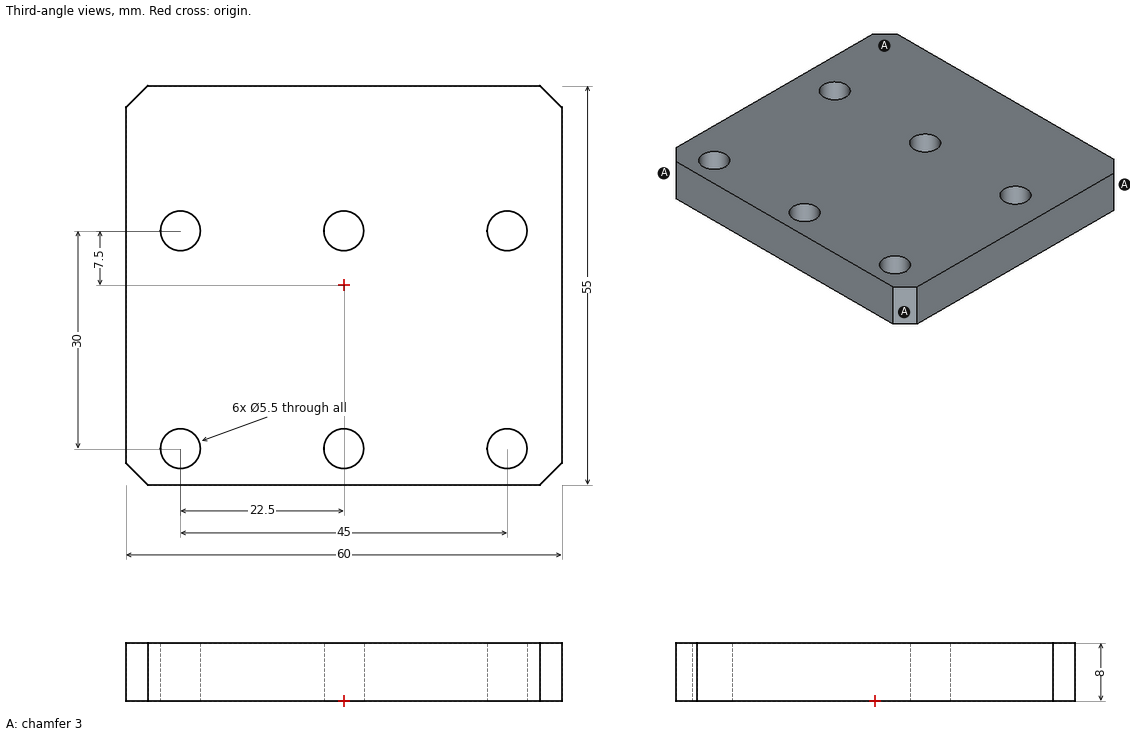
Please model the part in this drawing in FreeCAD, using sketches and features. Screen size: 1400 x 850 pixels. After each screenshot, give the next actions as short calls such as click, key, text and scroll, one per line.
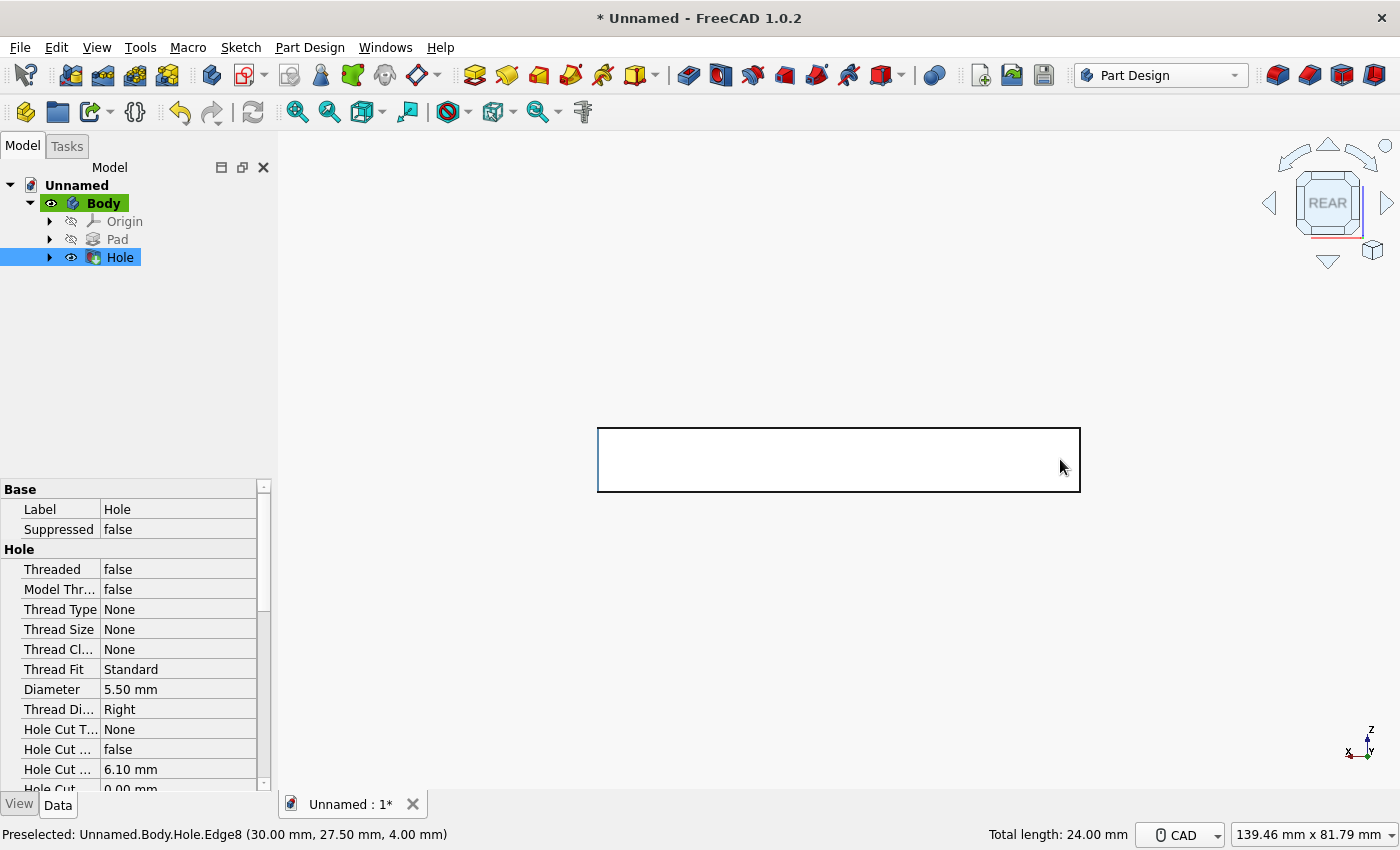
click(298, 112)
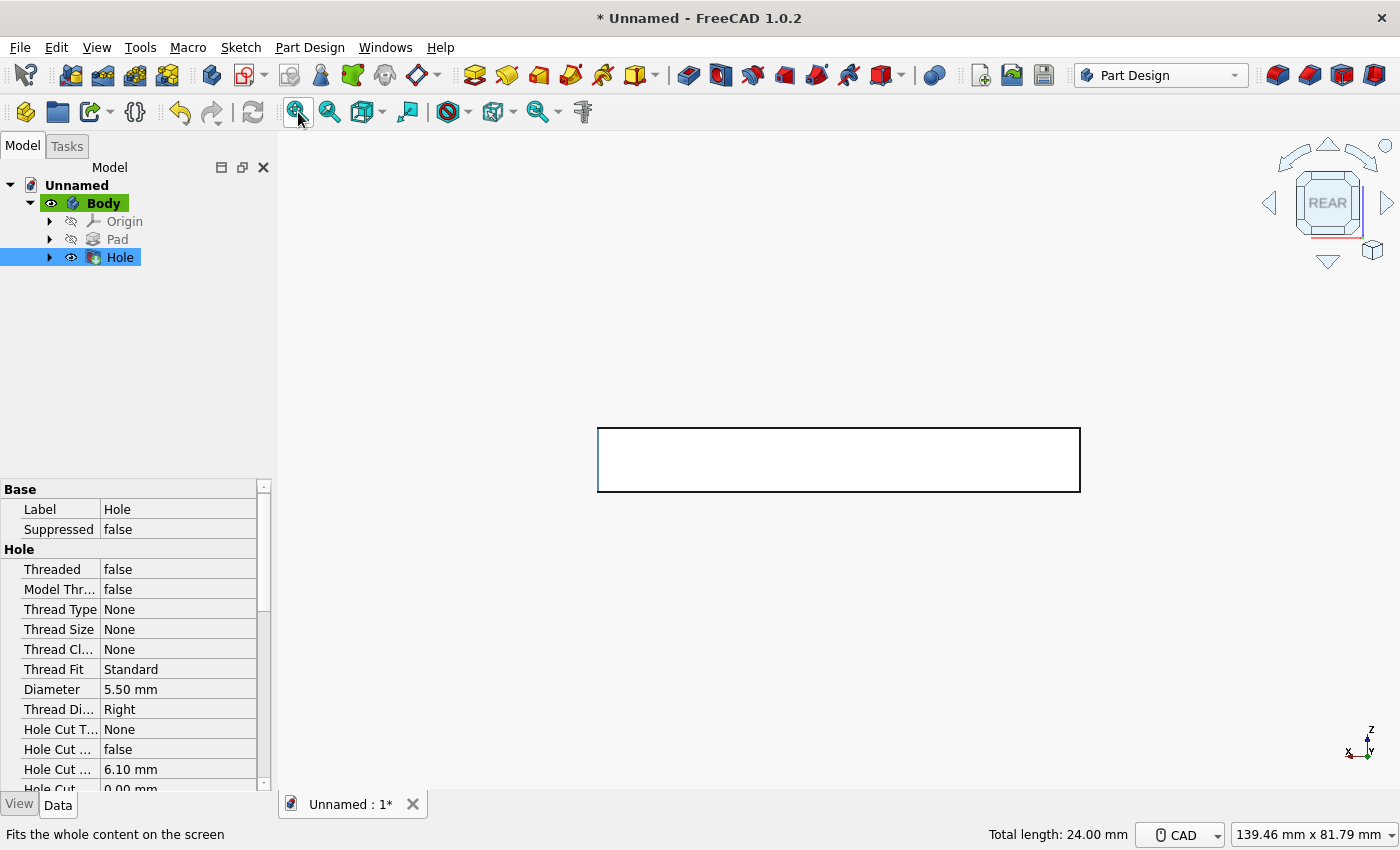
click(1080, 459, ctrl)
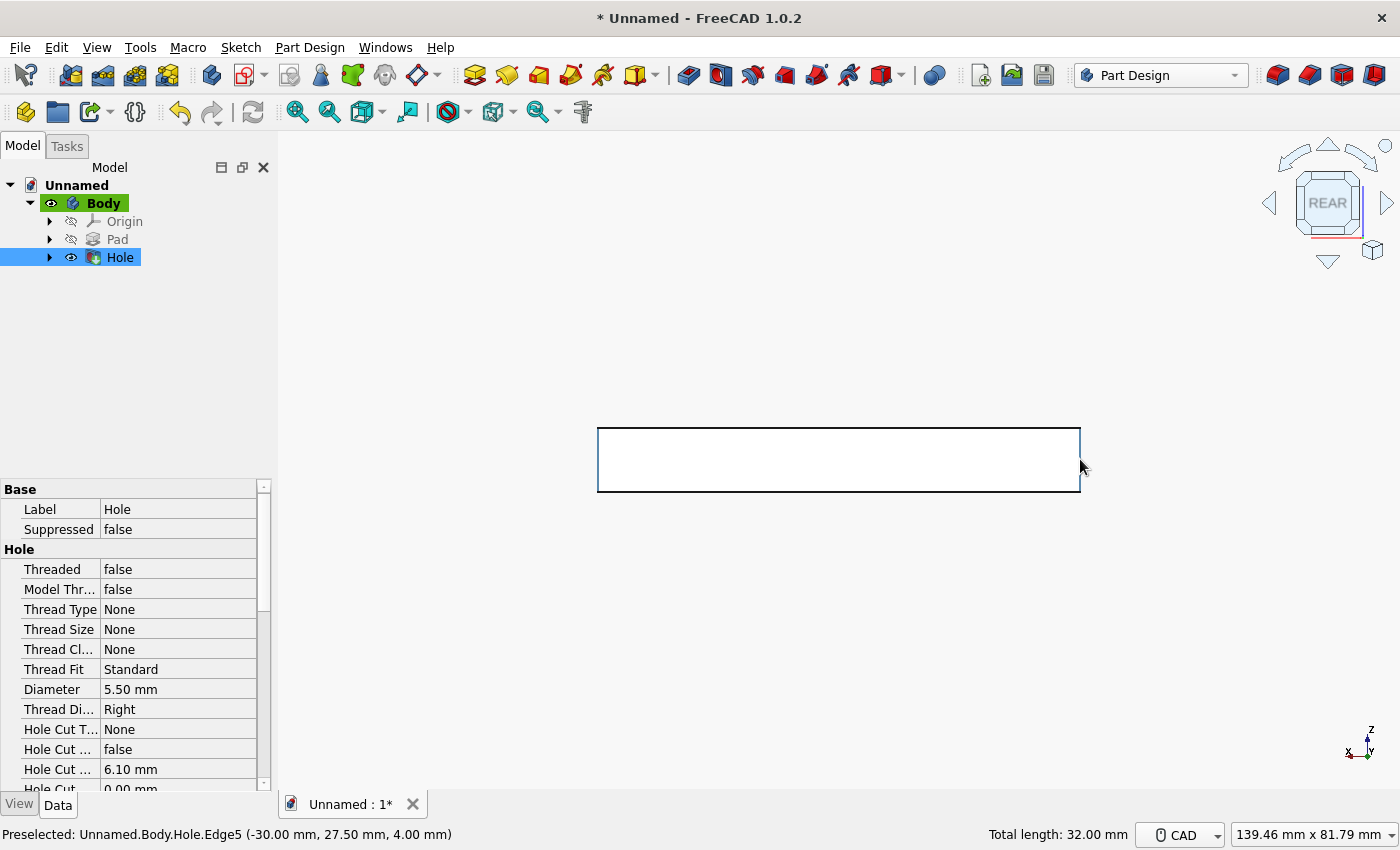
click(1310, 76)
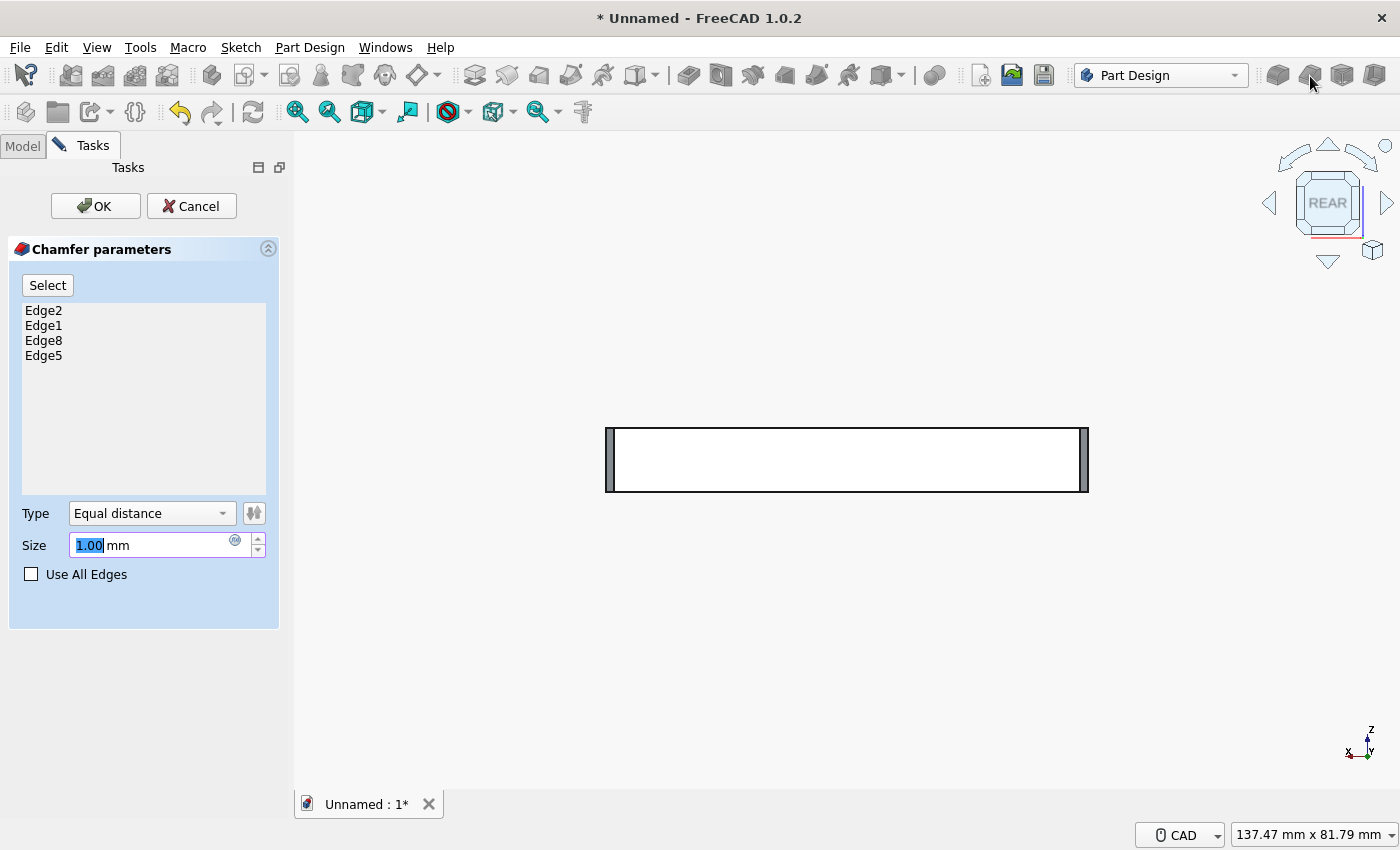
text(3)
key(Tab)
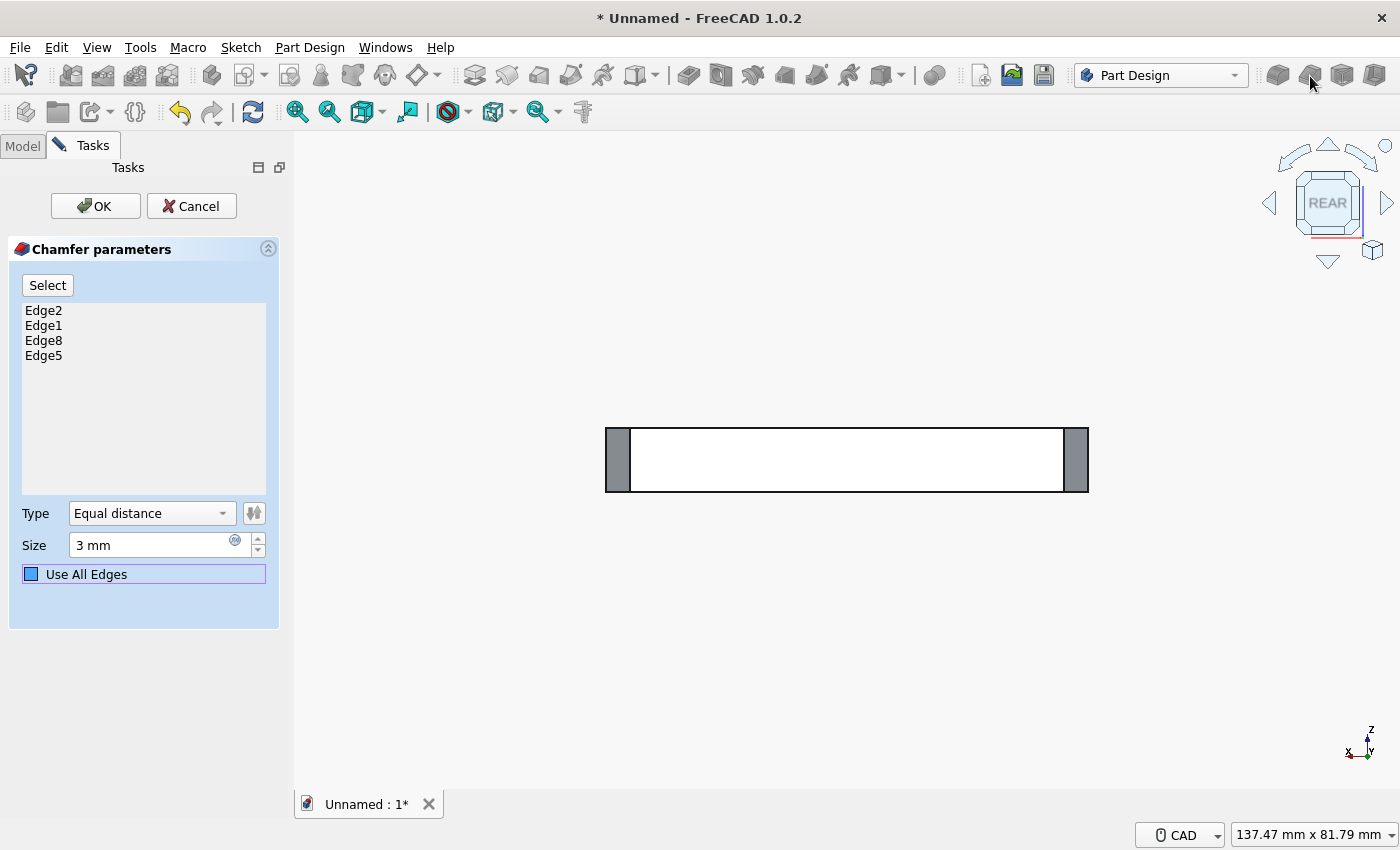
click(96, 206)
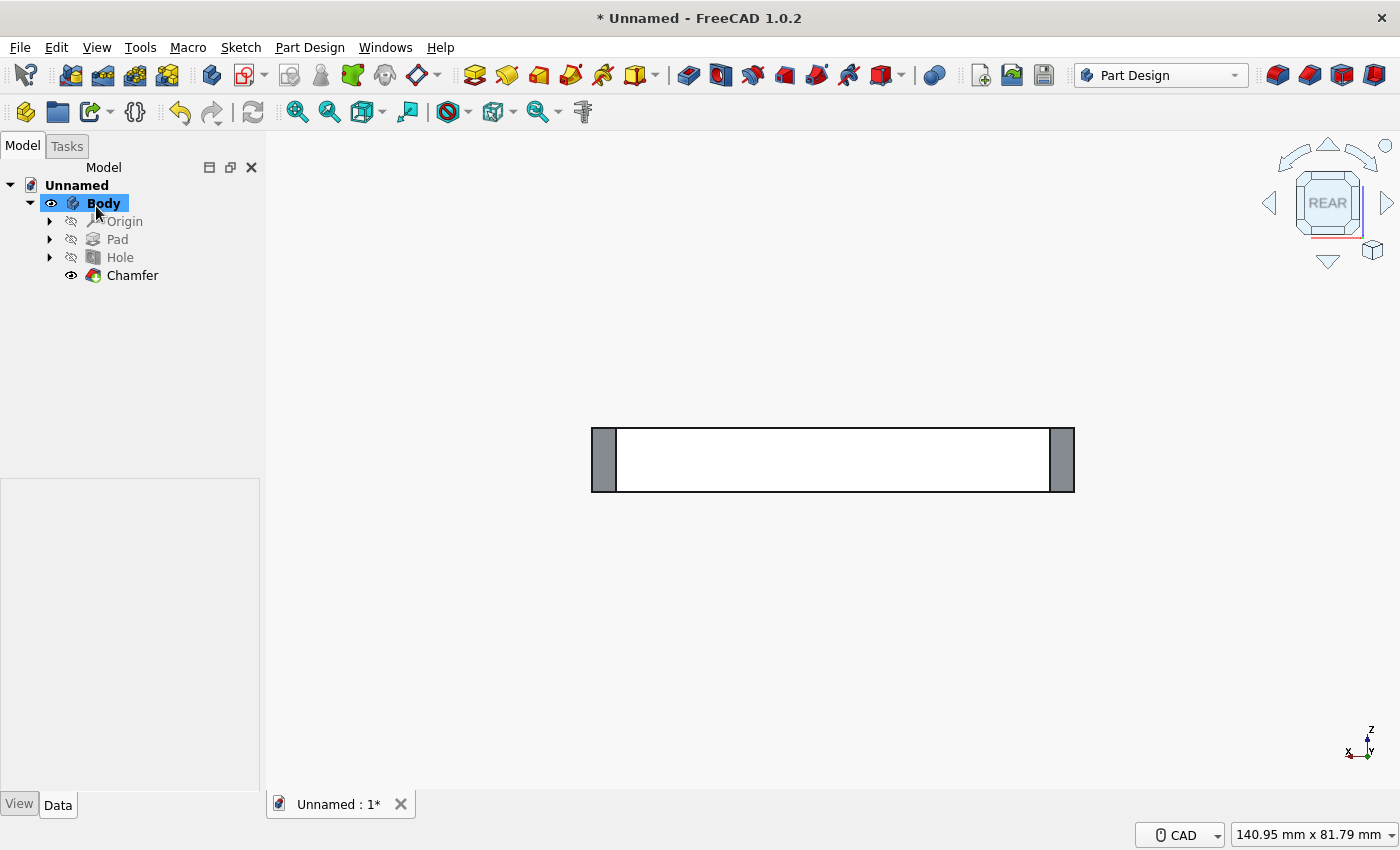
key(0)